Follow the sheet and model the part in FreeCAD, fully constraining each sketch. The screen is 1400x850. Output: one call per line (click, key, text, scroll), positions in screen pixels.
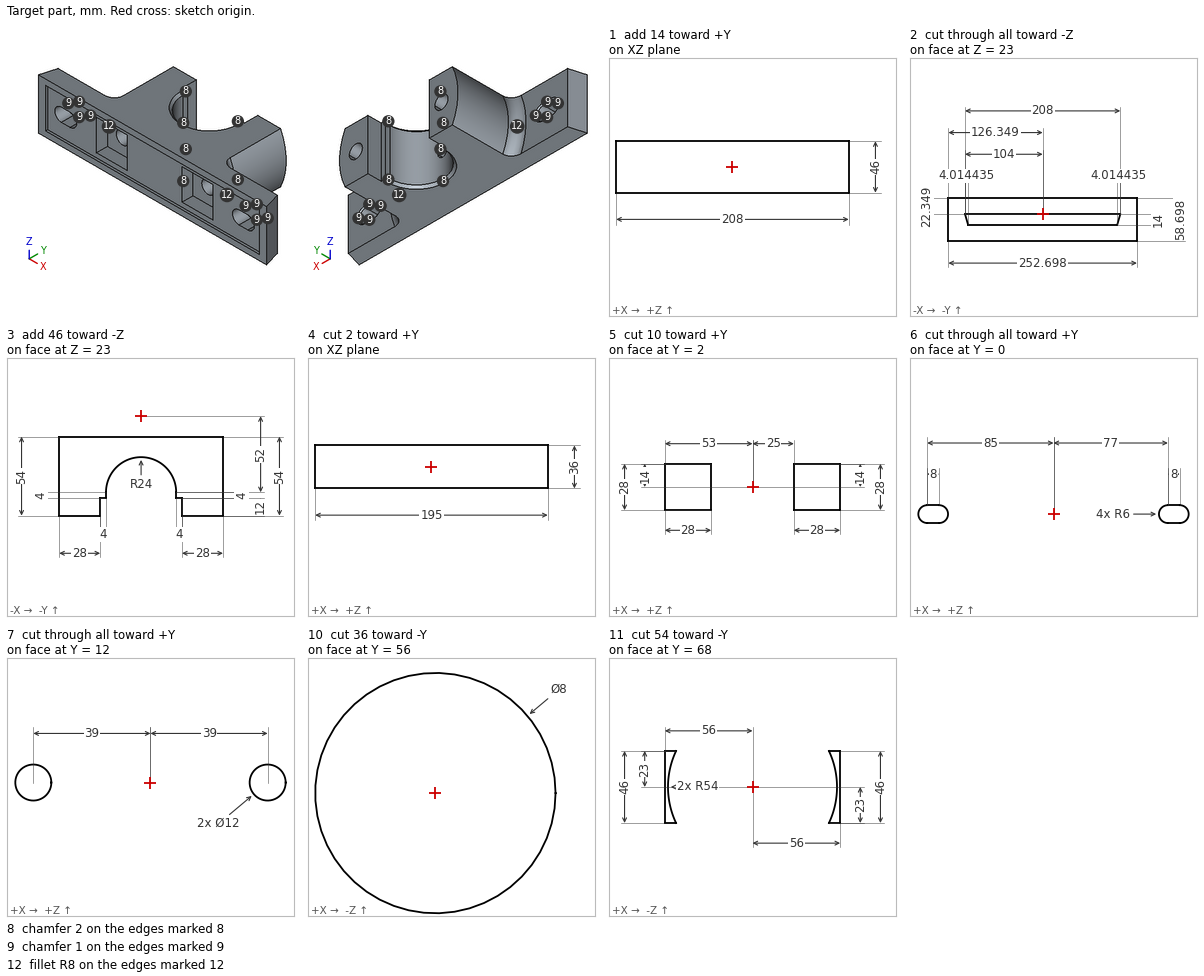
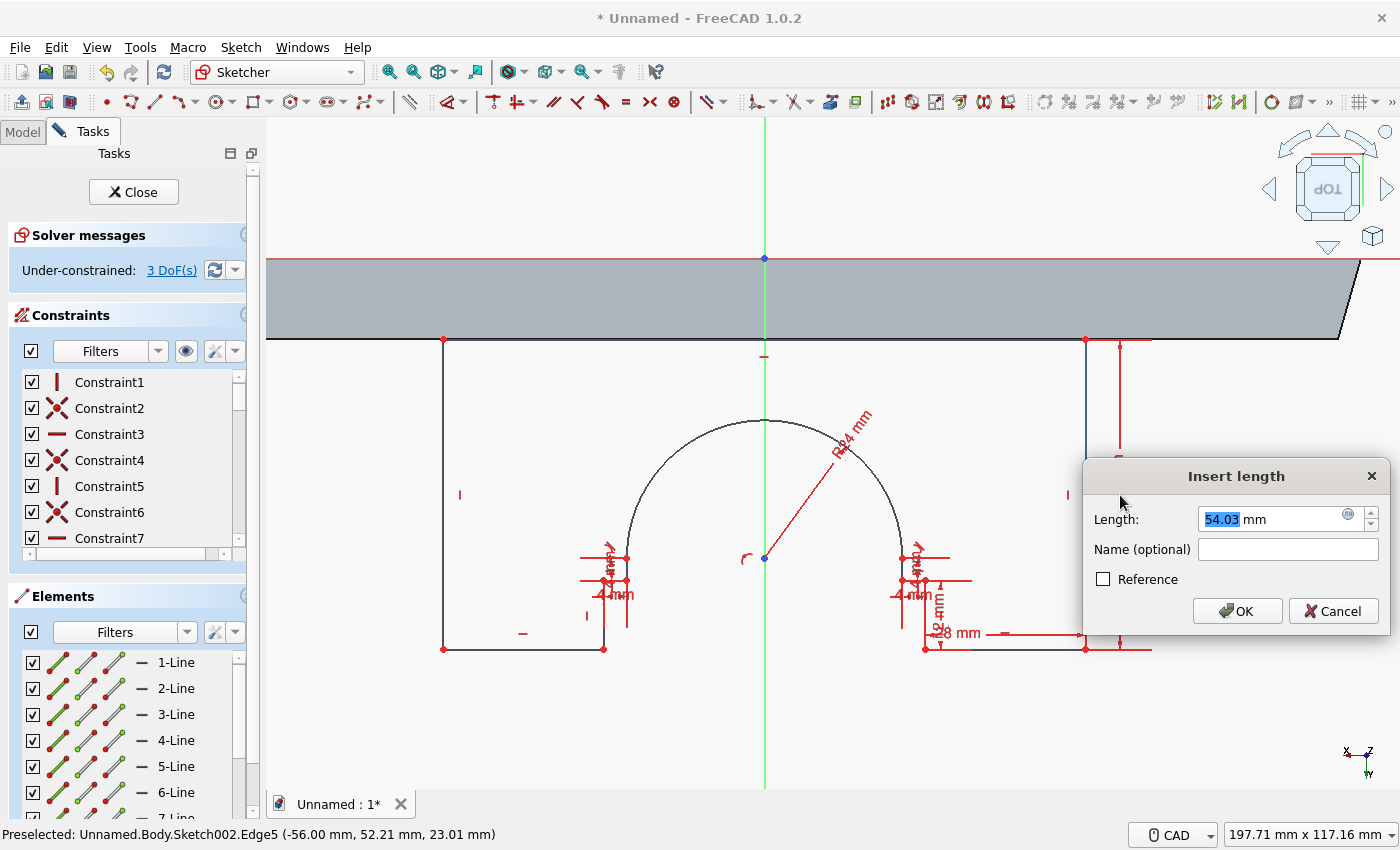
text(54)
key(Return)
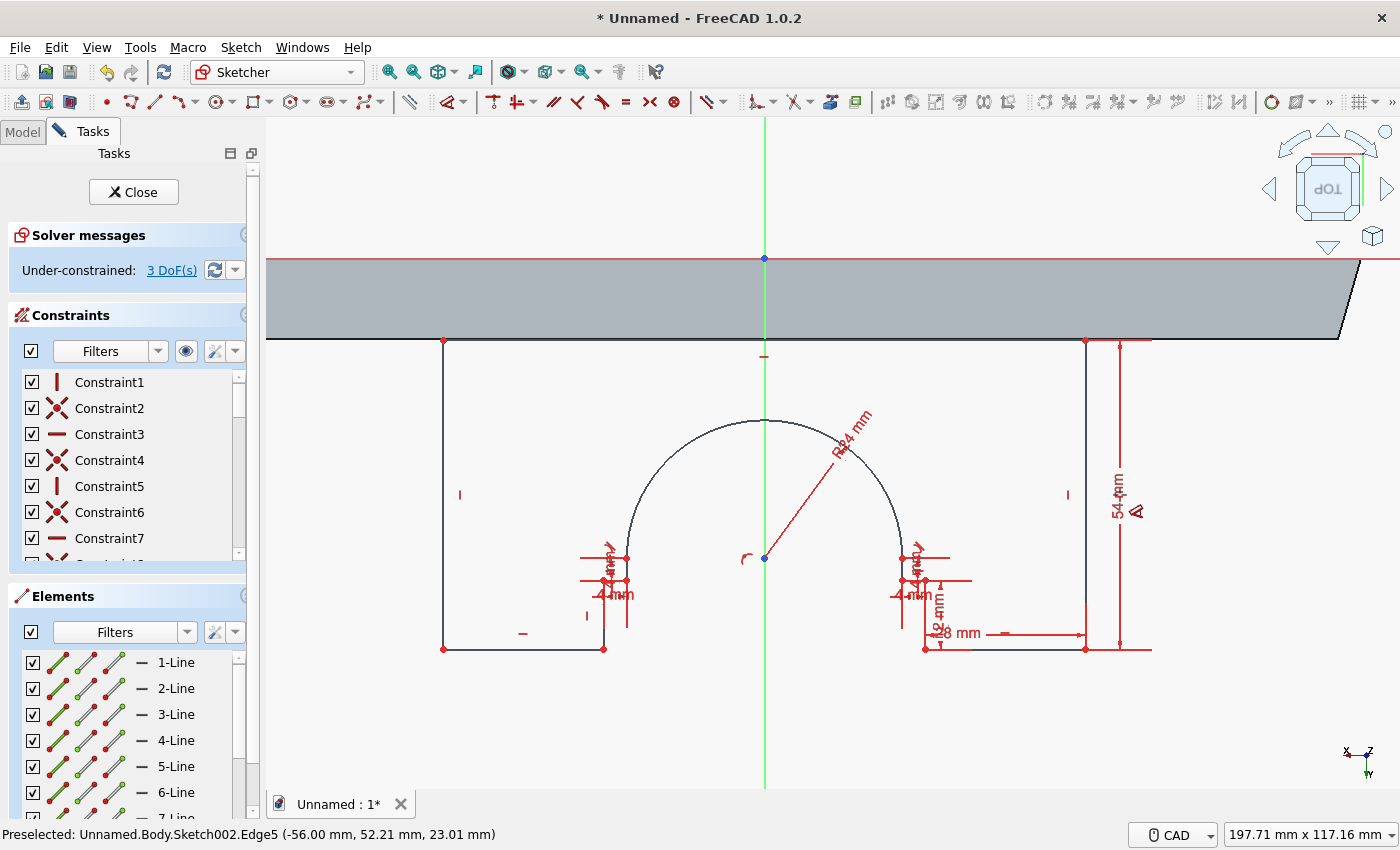
click(443, 433)
click(409, 495)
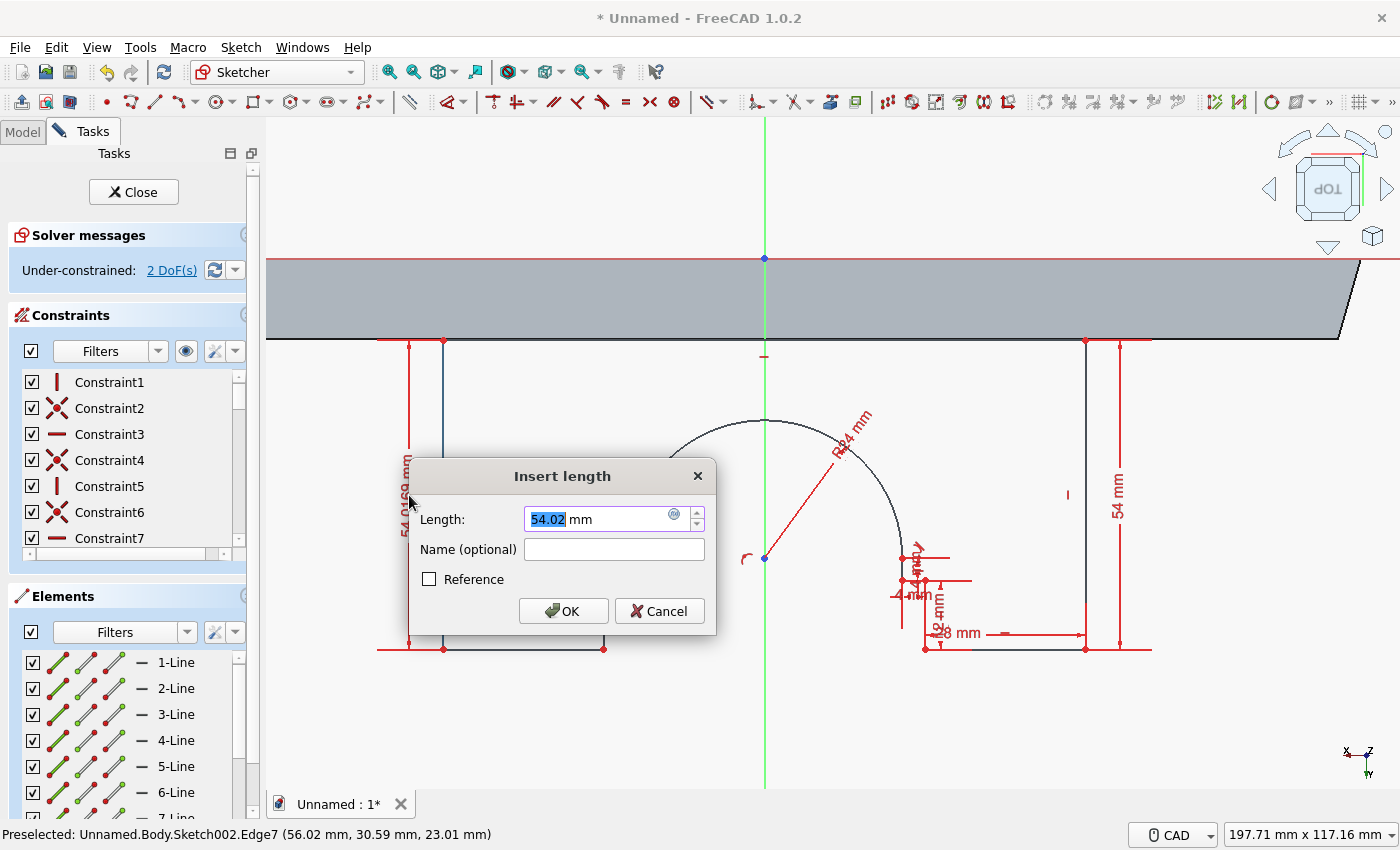
text(54)
key(Return)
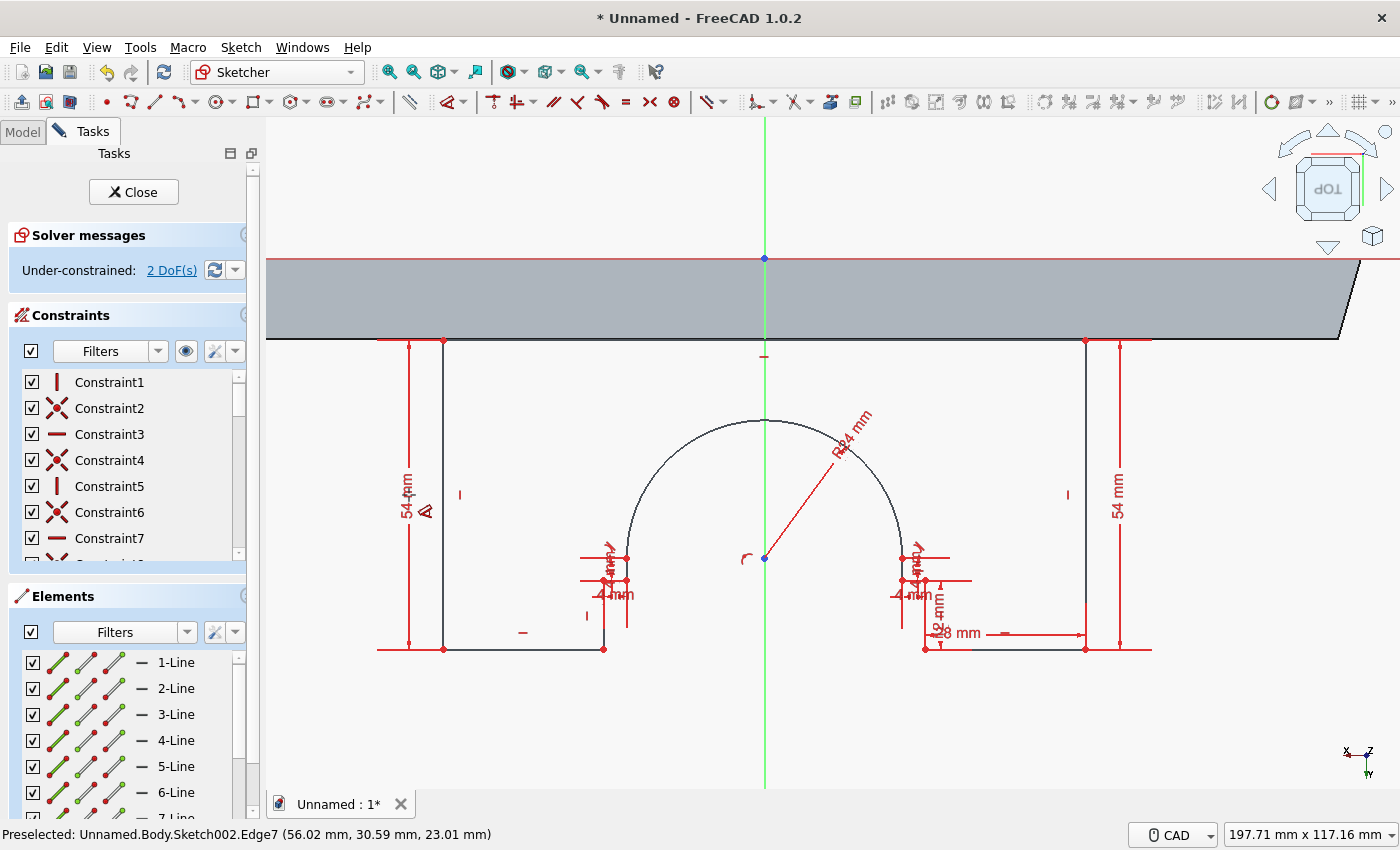
click(491, 650)
click(524, 684)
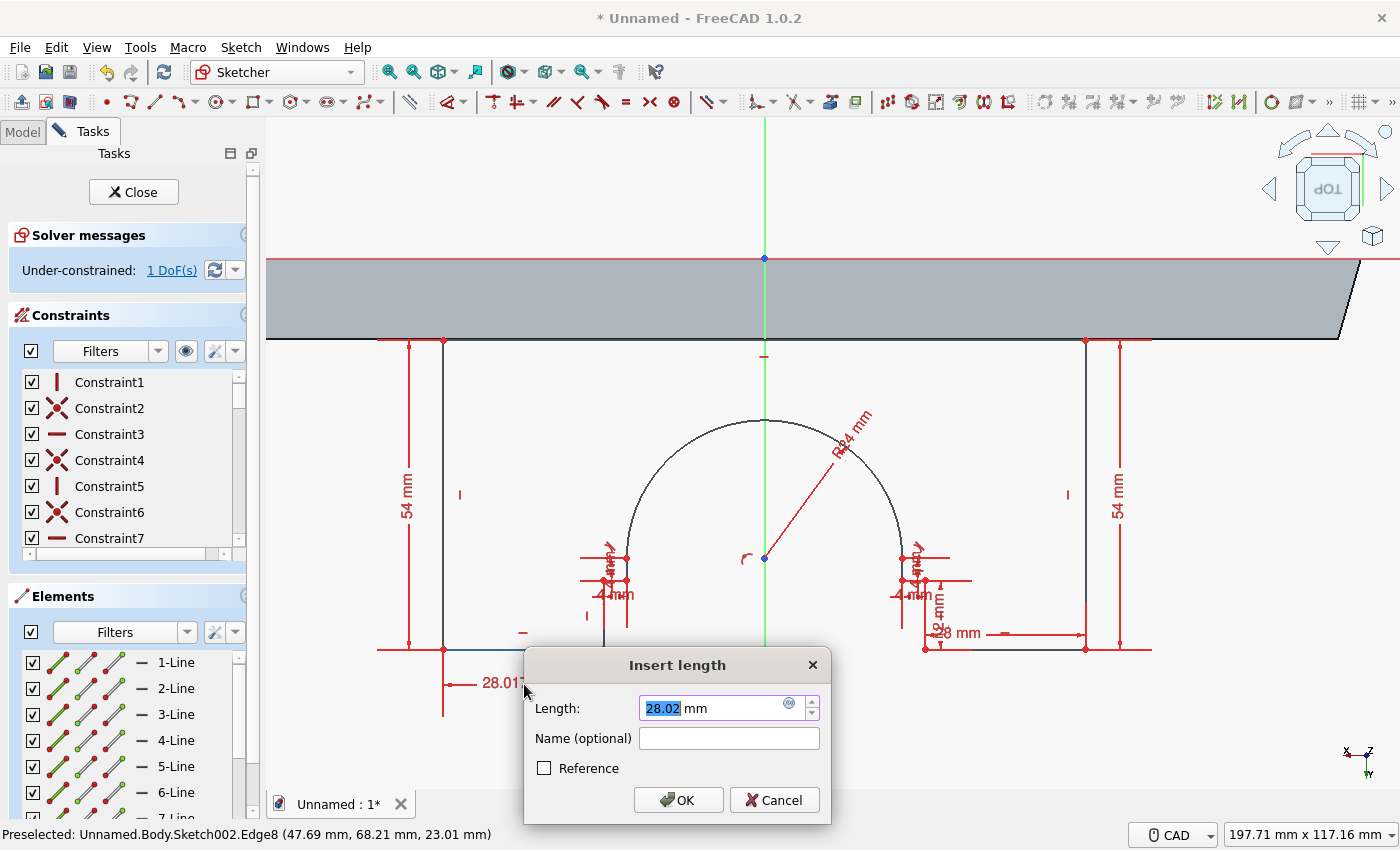
text(28)
key(Return)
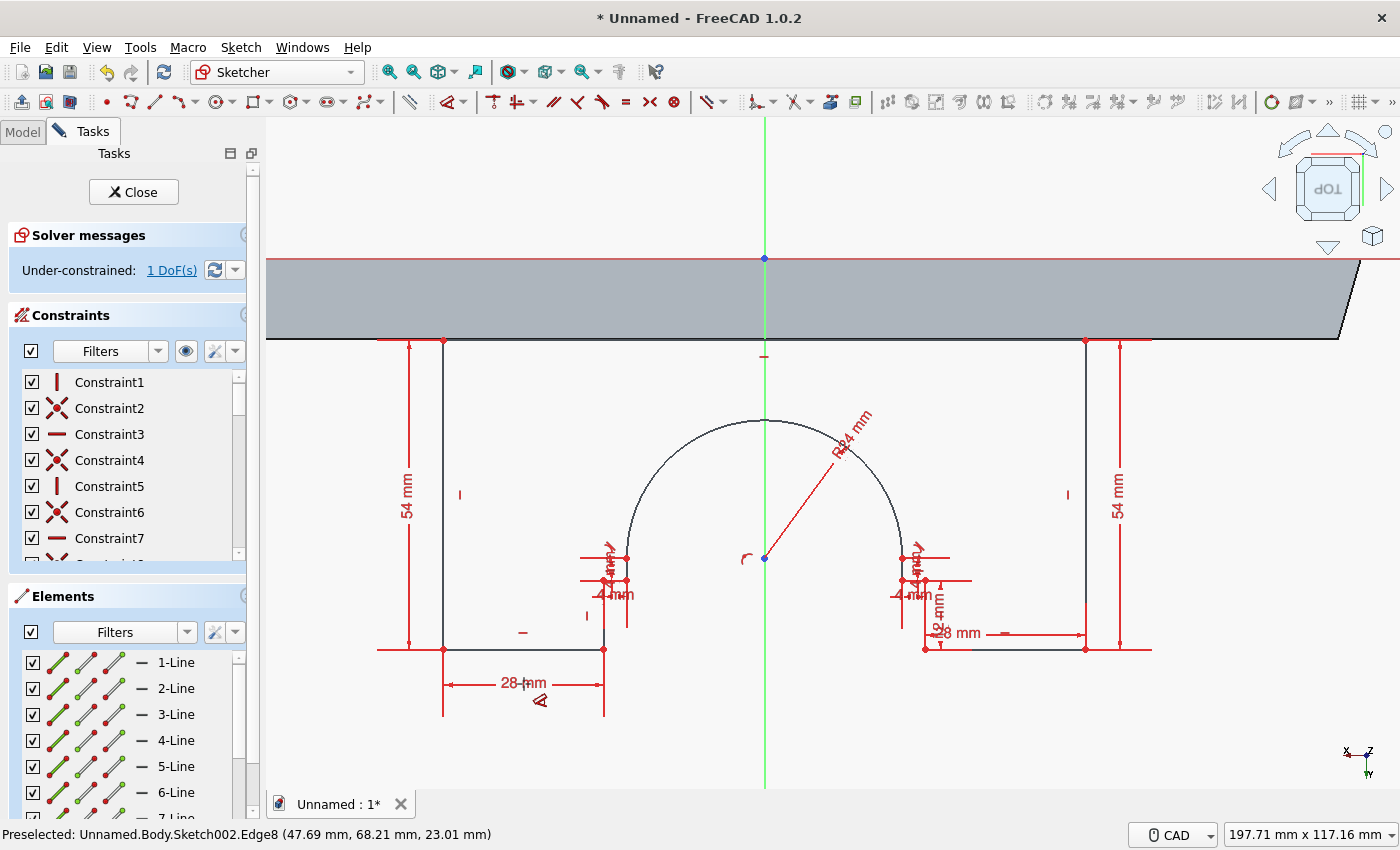
click(902, 558)
click(936, 408)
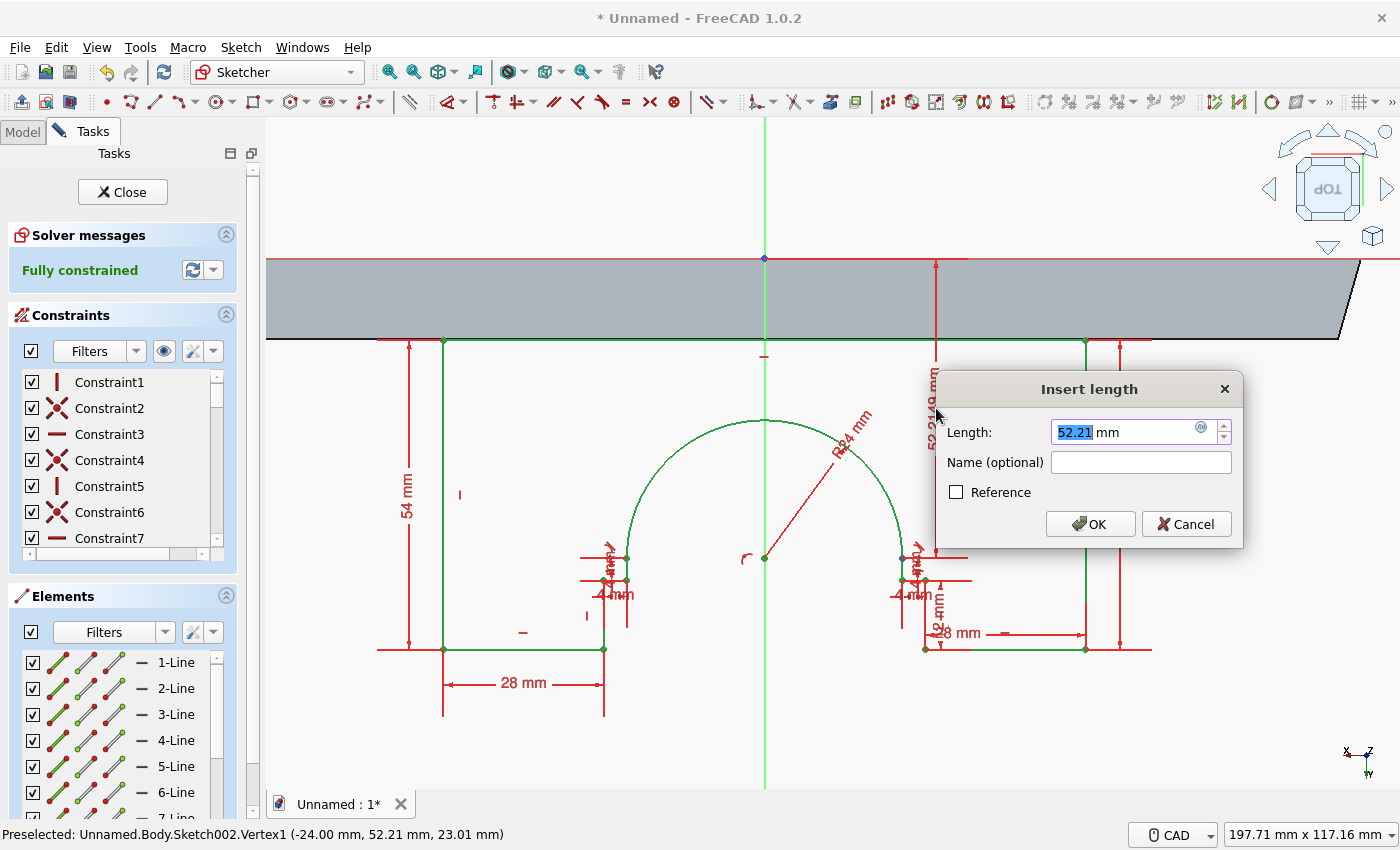
text(52)
key(Return)
key(Escape)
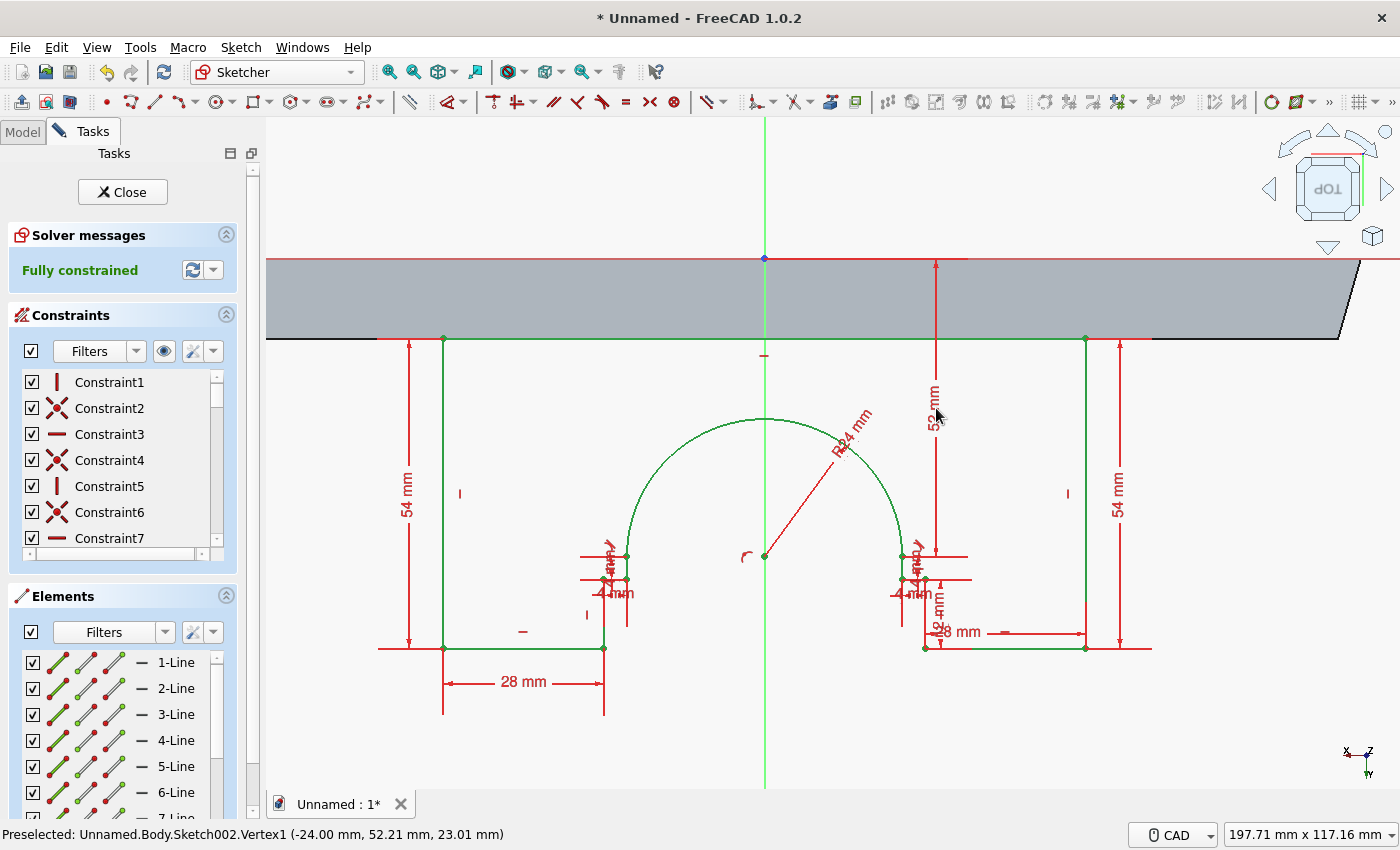
click(123, 192)